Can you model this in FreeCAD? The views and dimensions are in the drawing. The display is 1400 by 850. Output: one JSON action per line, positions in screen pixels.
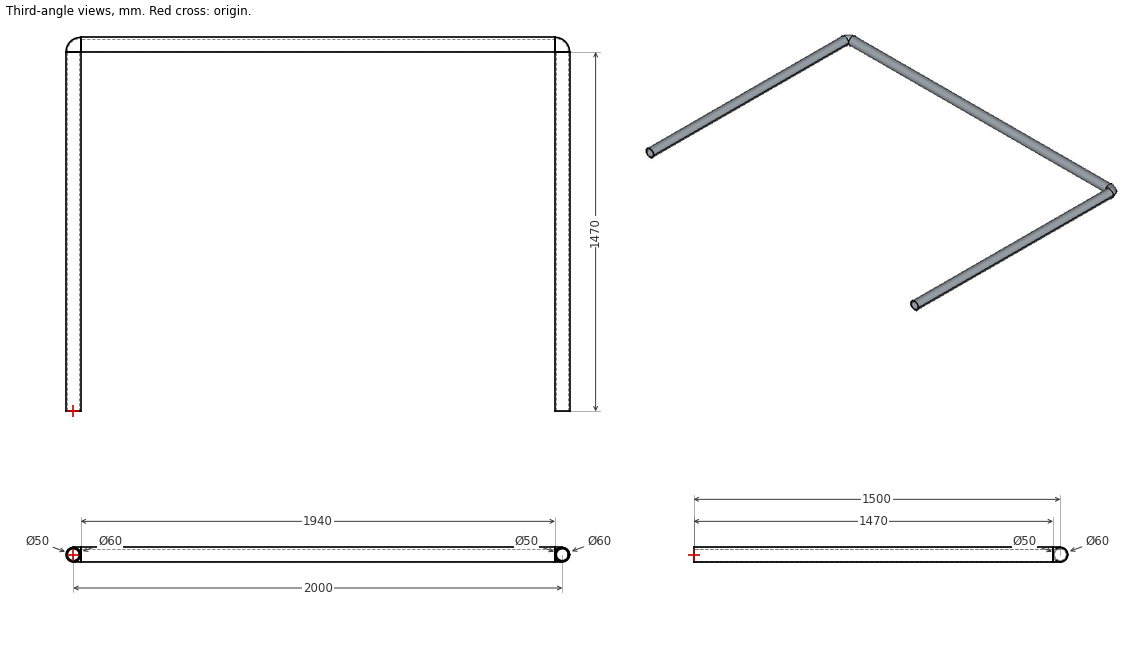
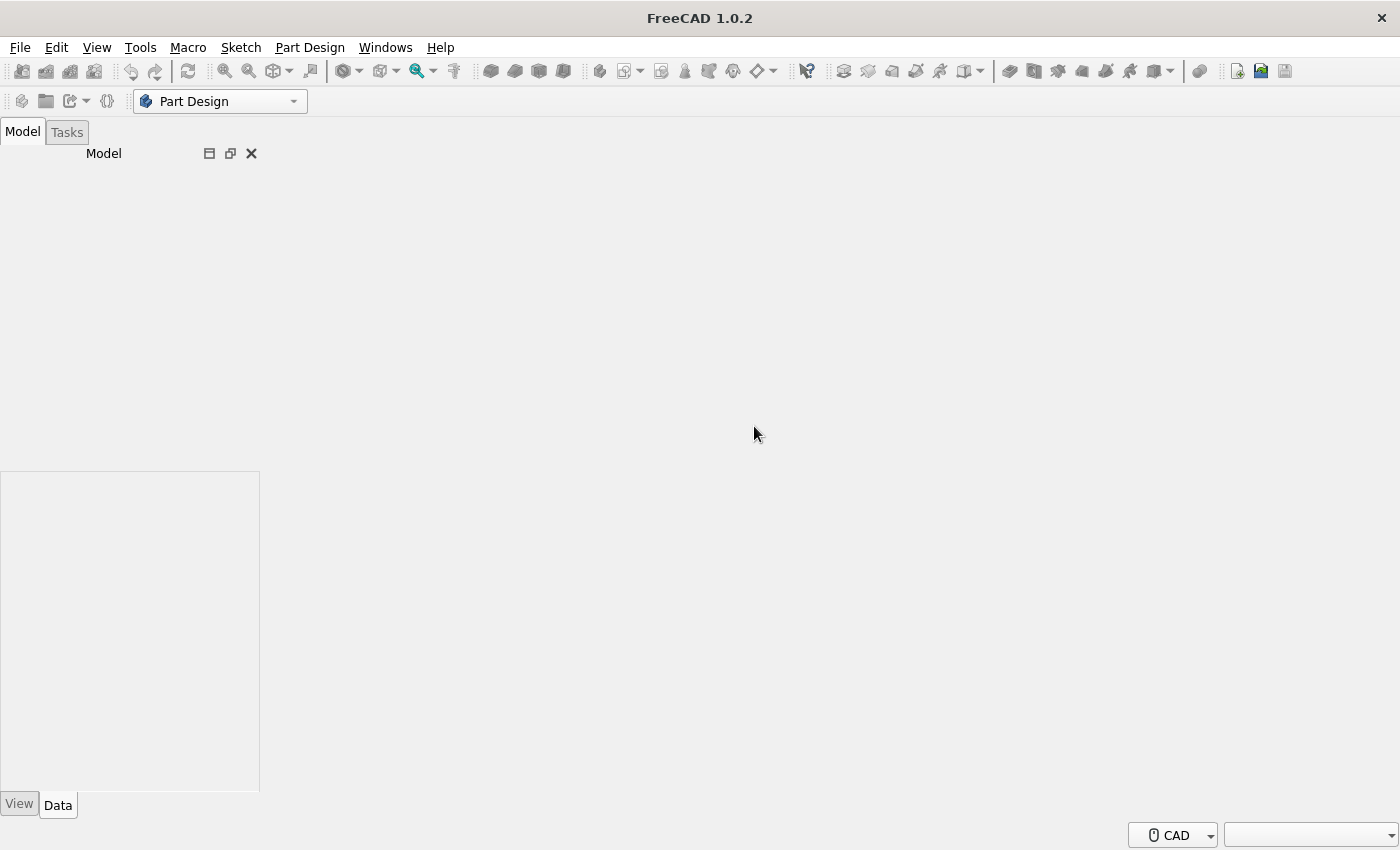
{"action": "key", "text": "ctrl+n"}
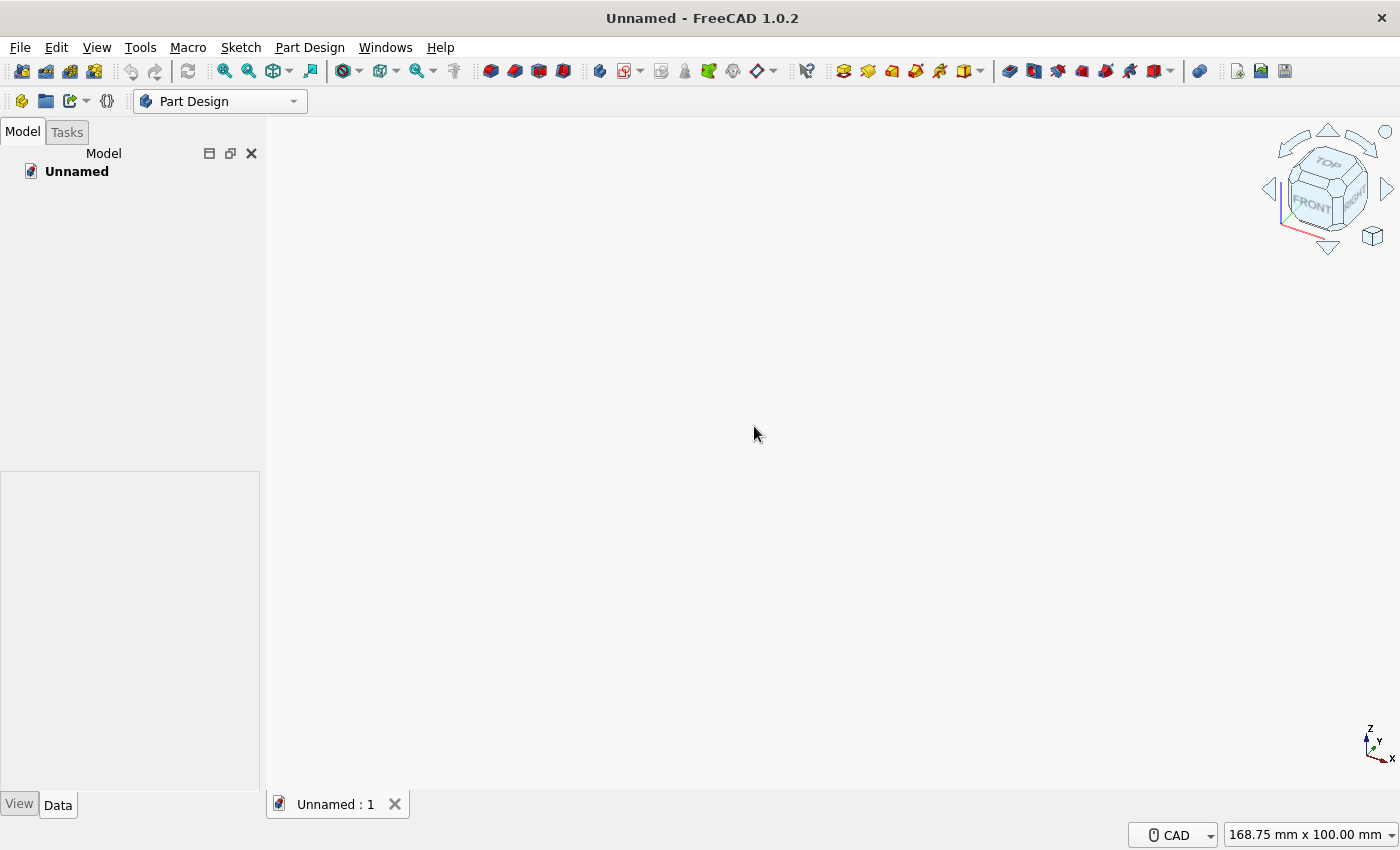
{"action": "left_click", "coordinate": [624, 72]}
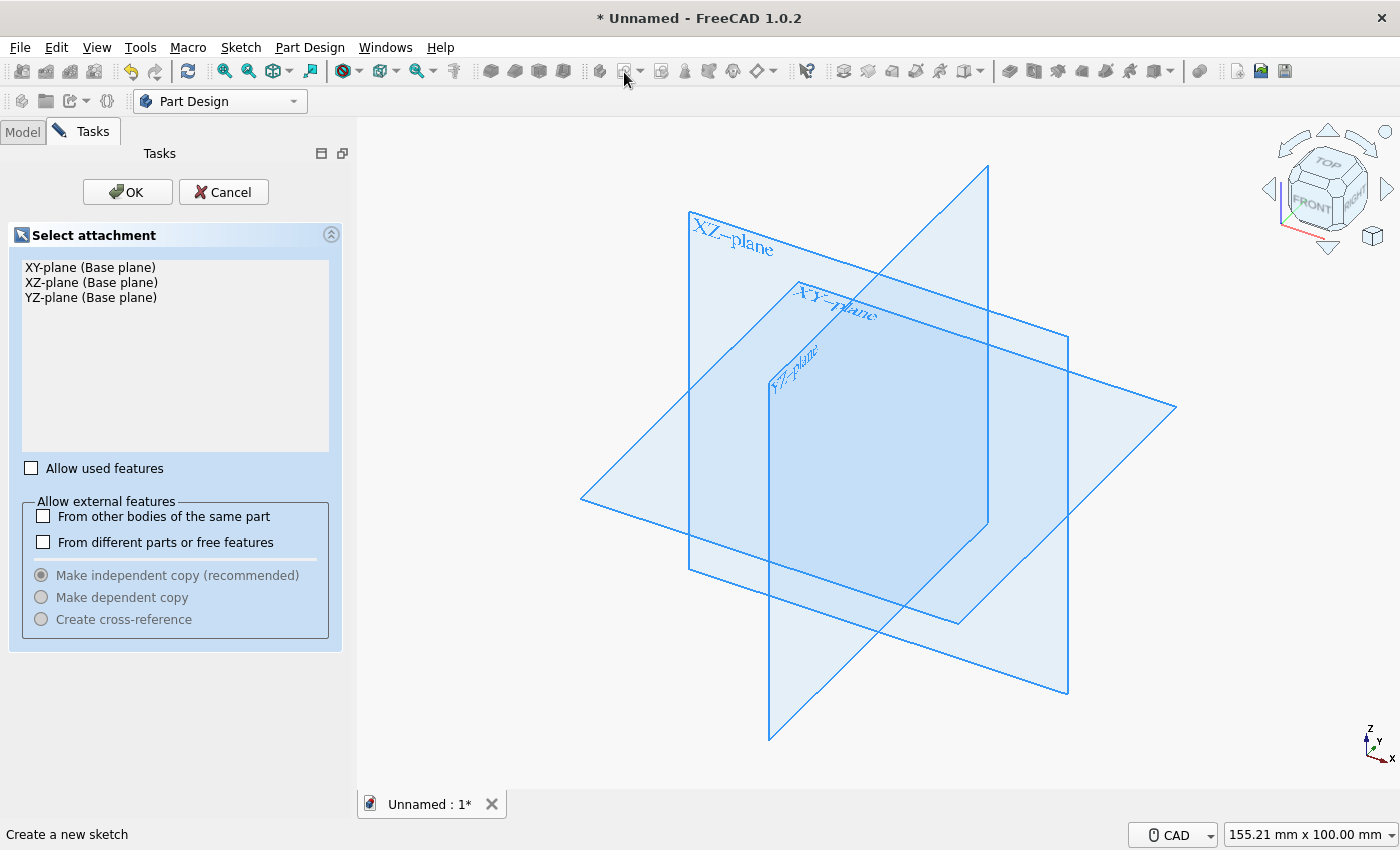
{"action": "left_click", "coordinate": [82, 282]}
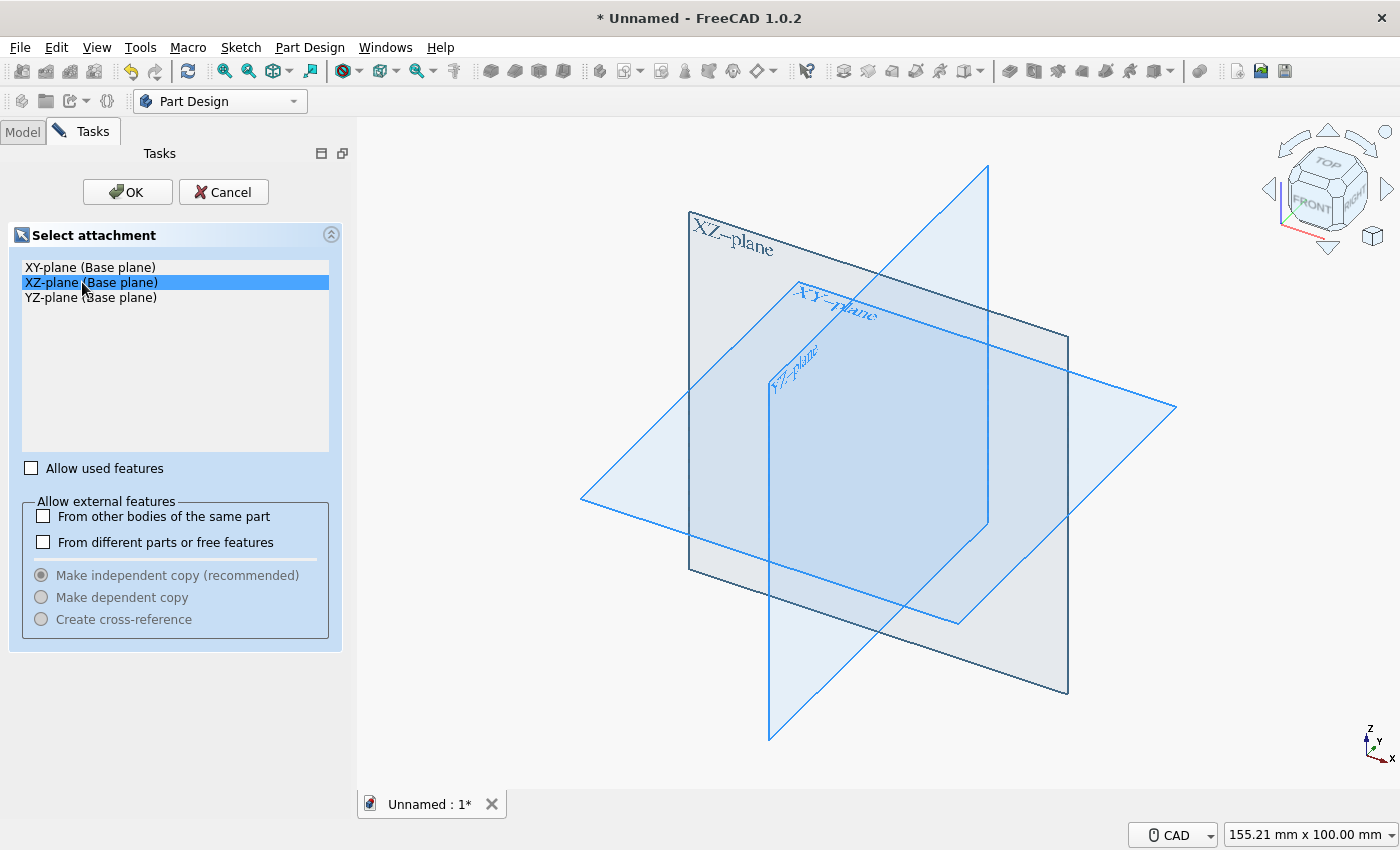
{"action": "left_click", "coordinate": [128, 192]}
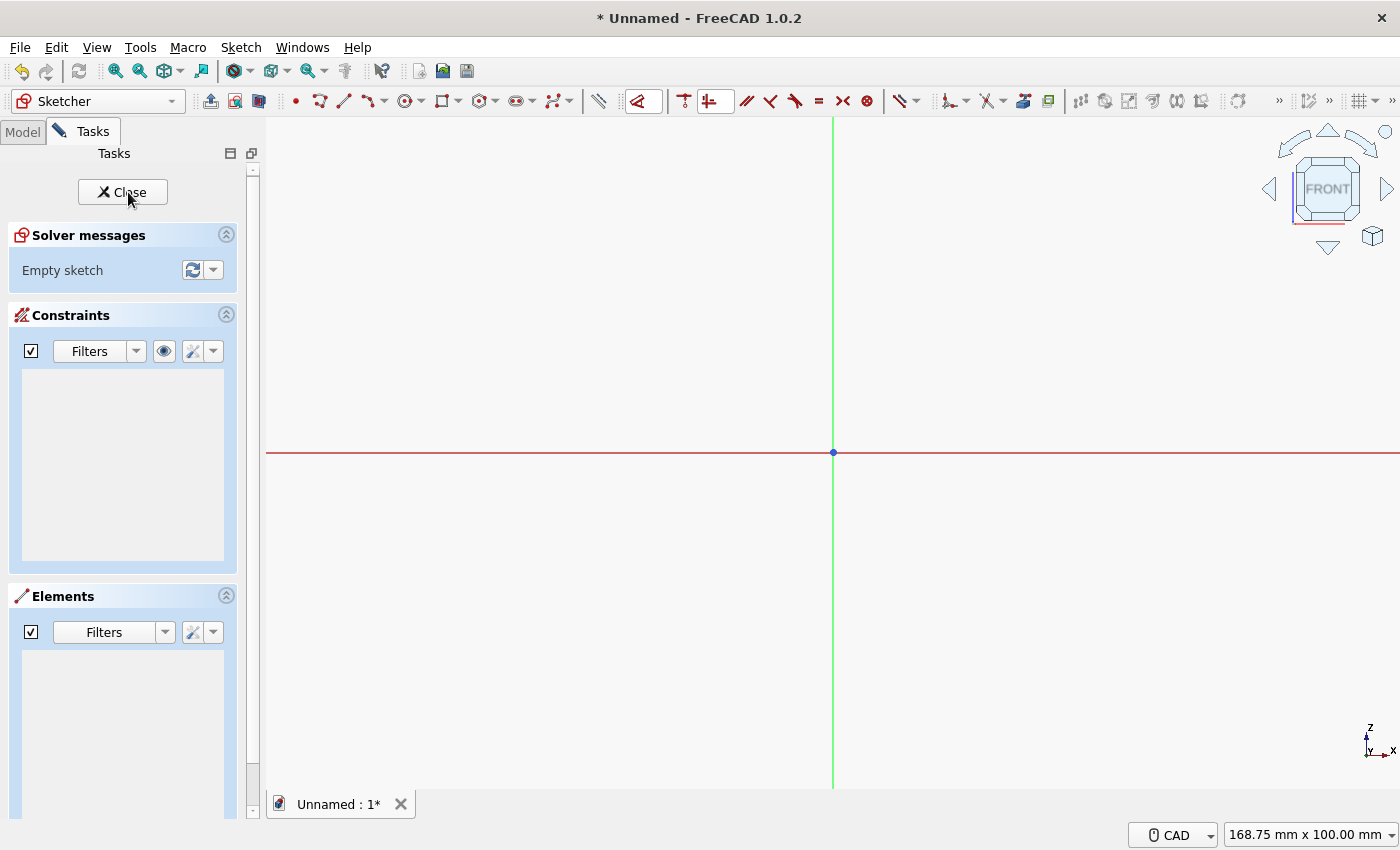
{"action": "left_click", "coordinate": [406, 102]}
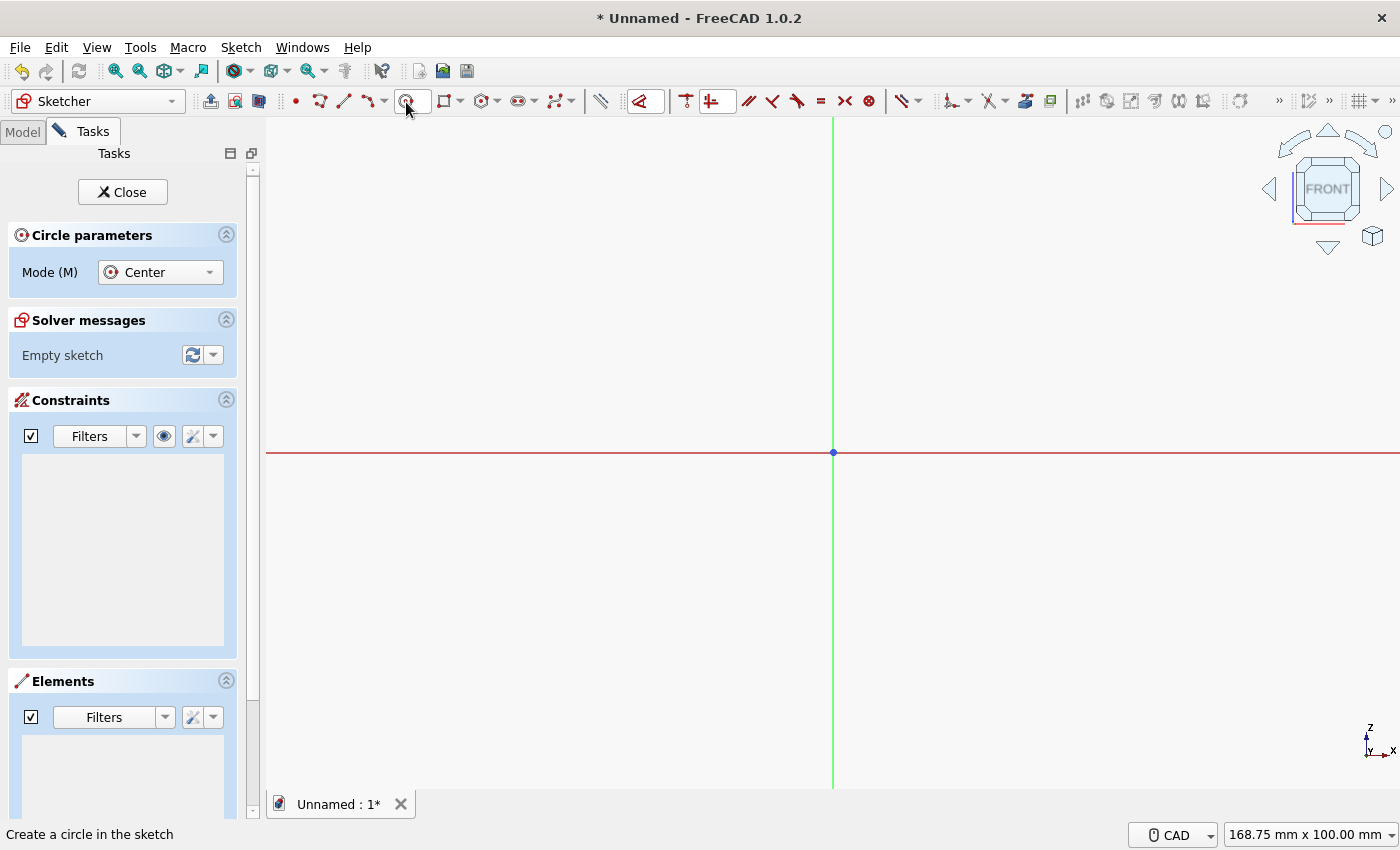
{"action": "left_click", "coordinate": [833, 453]}
{"action": "mouse_move", "coordinate": [976, 310]}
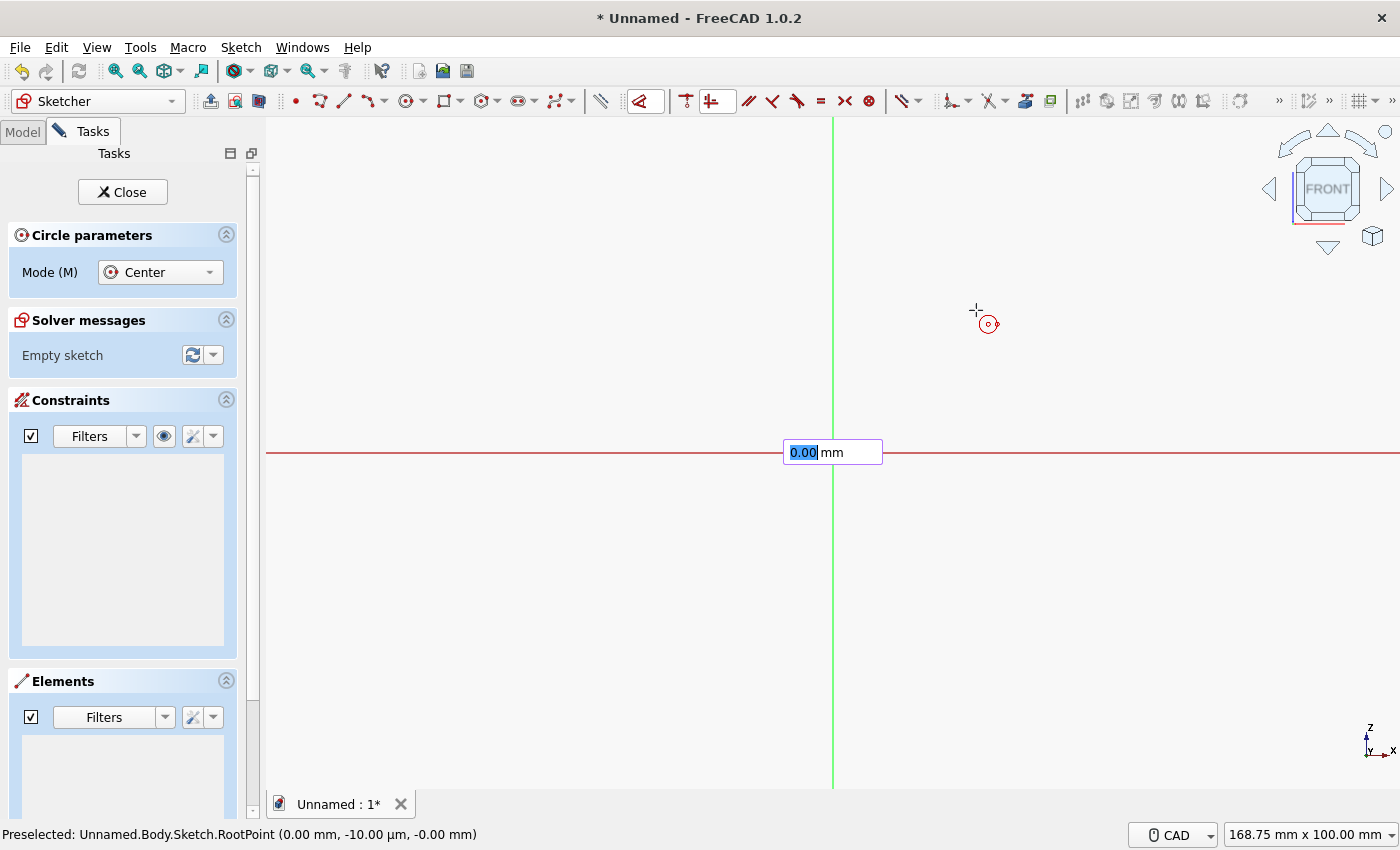
{"action": "type", "text": "60"}
{"action": "key", "text": "Return"}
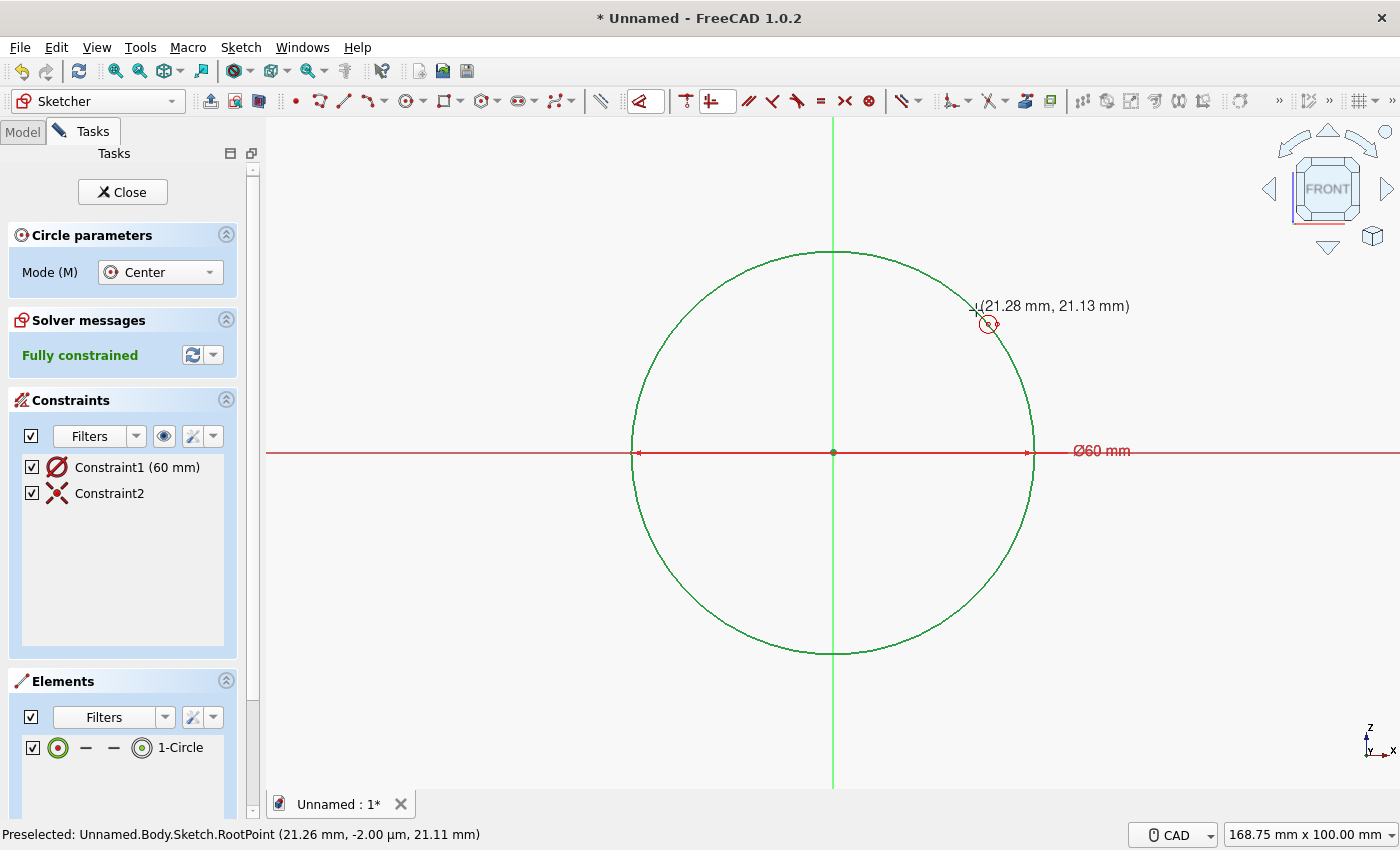
{"action": "left_click", "coordinate": [833, 453]}
{"action": "mouse_move", "coordinate": [952, 334]}